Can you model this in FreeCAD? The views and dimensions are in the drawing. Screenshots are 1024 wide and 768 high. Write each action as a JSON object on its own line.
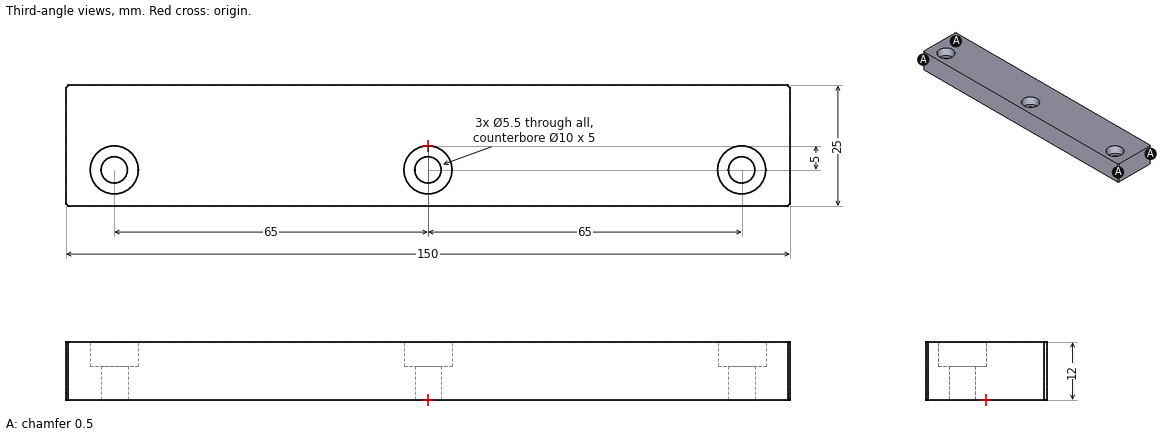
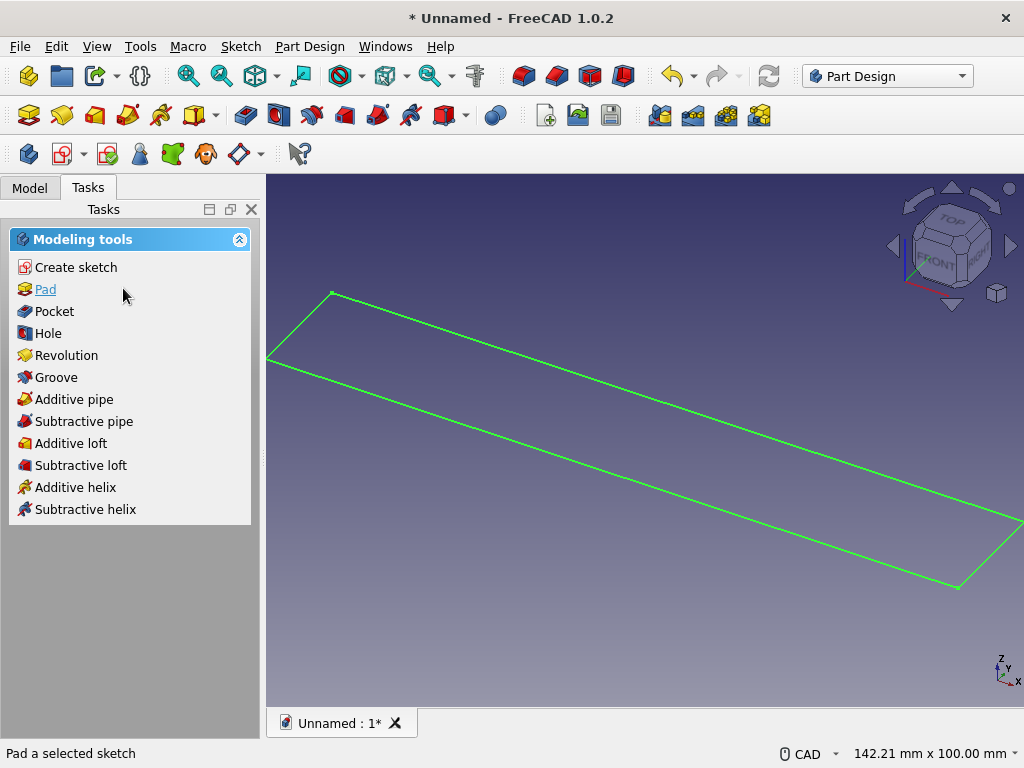
{"action": "left_click", "coordinate": [29, 116]}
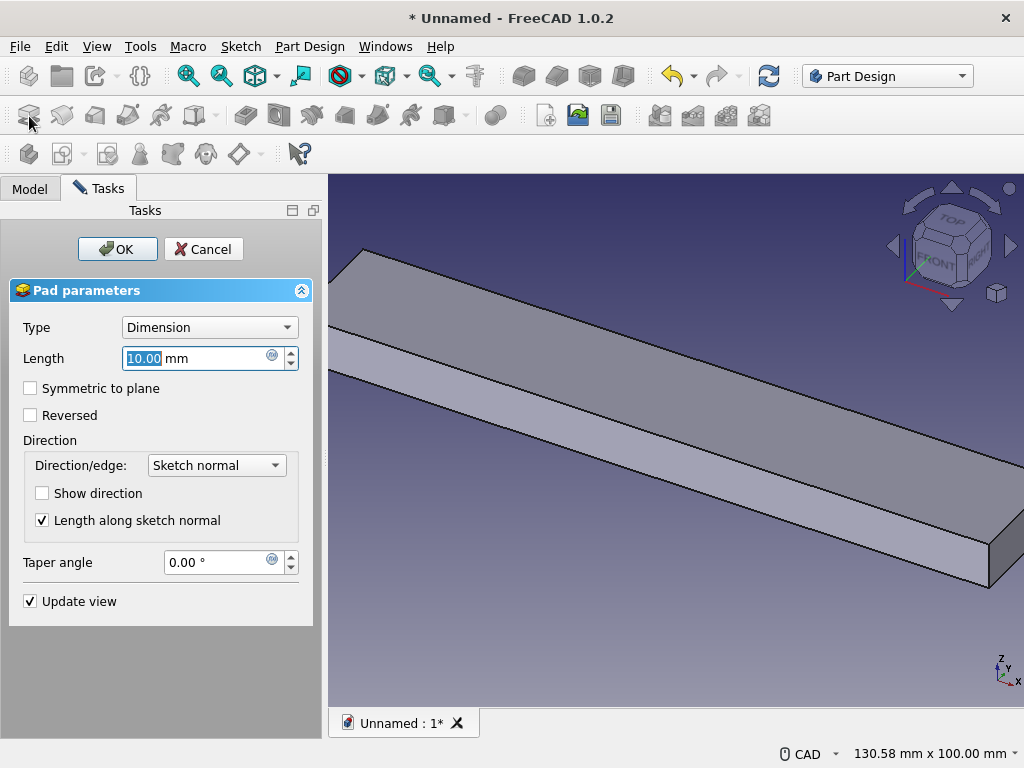
{"action": "type", "text": "12"}
{"action": "key", "text": "Tab"}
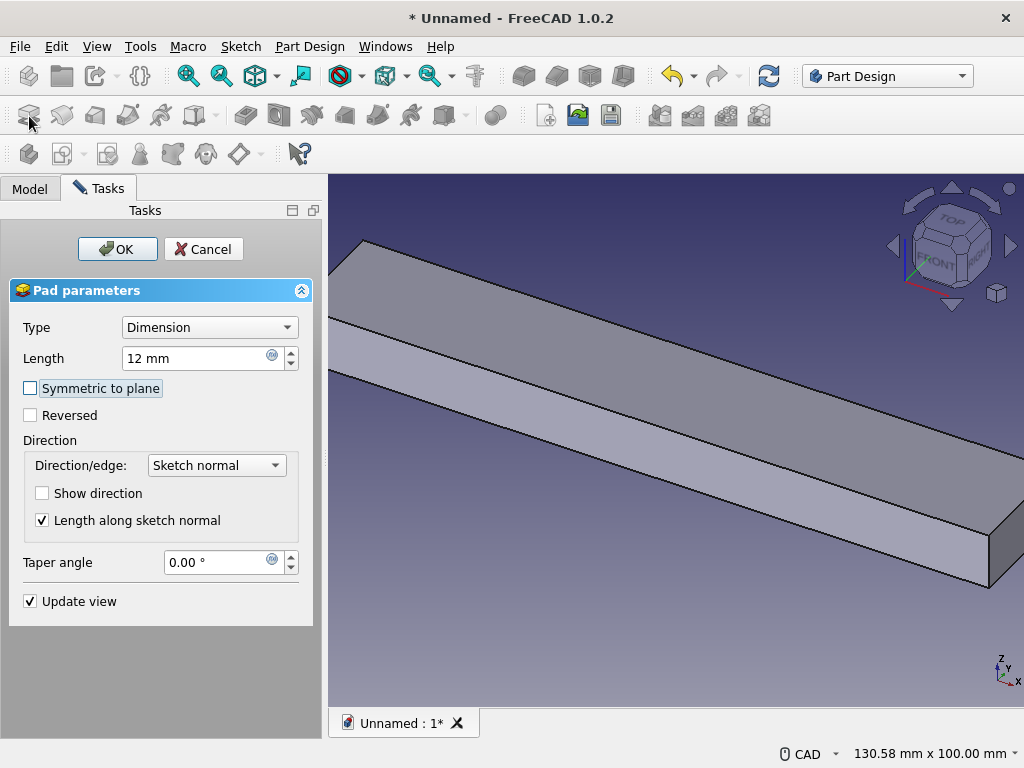
{"action": "left_click", "coordinate": [118, 249]}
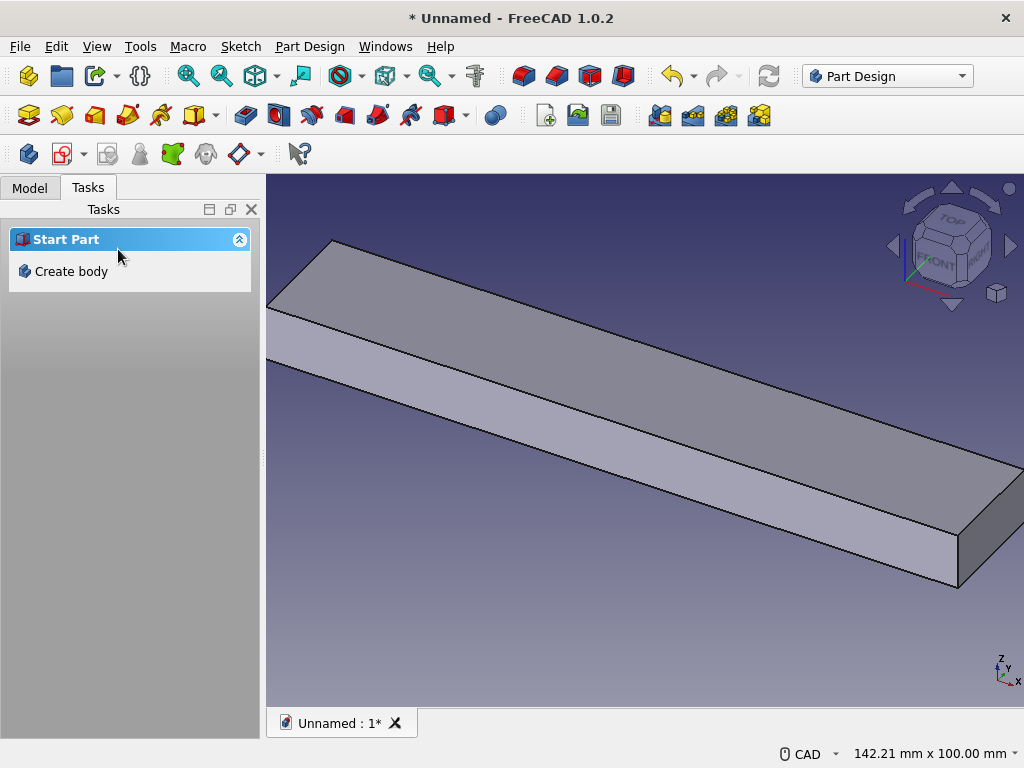
{"action": "left_click", "coordinate": [189, 76]}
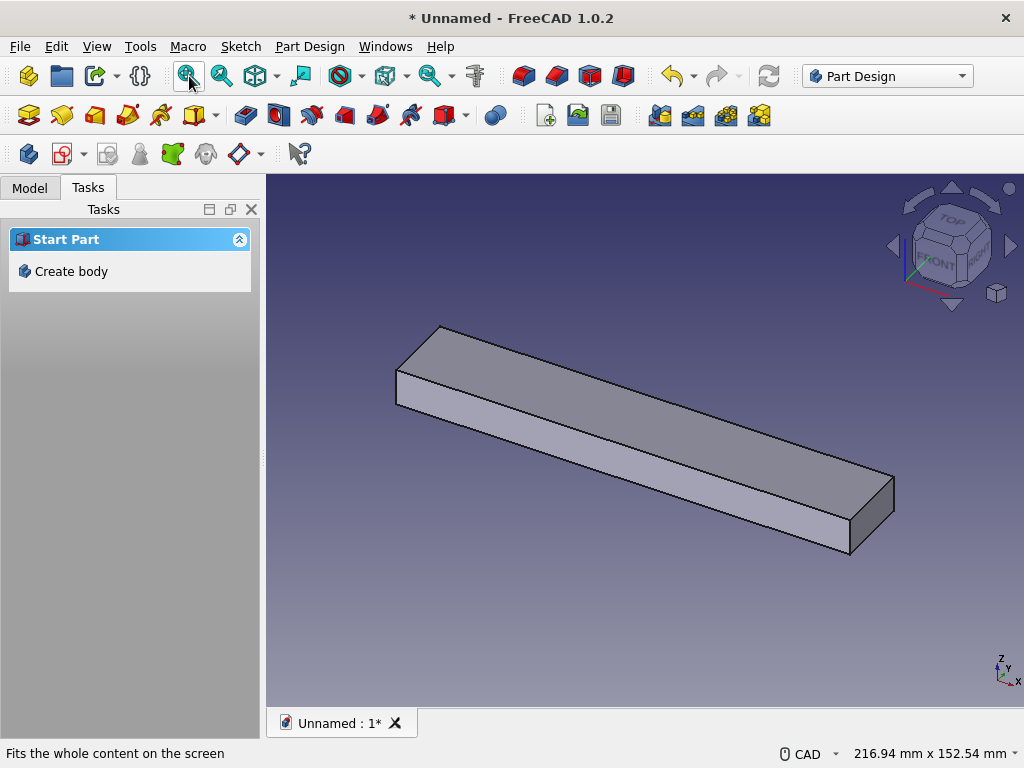
{"action": "left_click", "coordinate": [775, 465]}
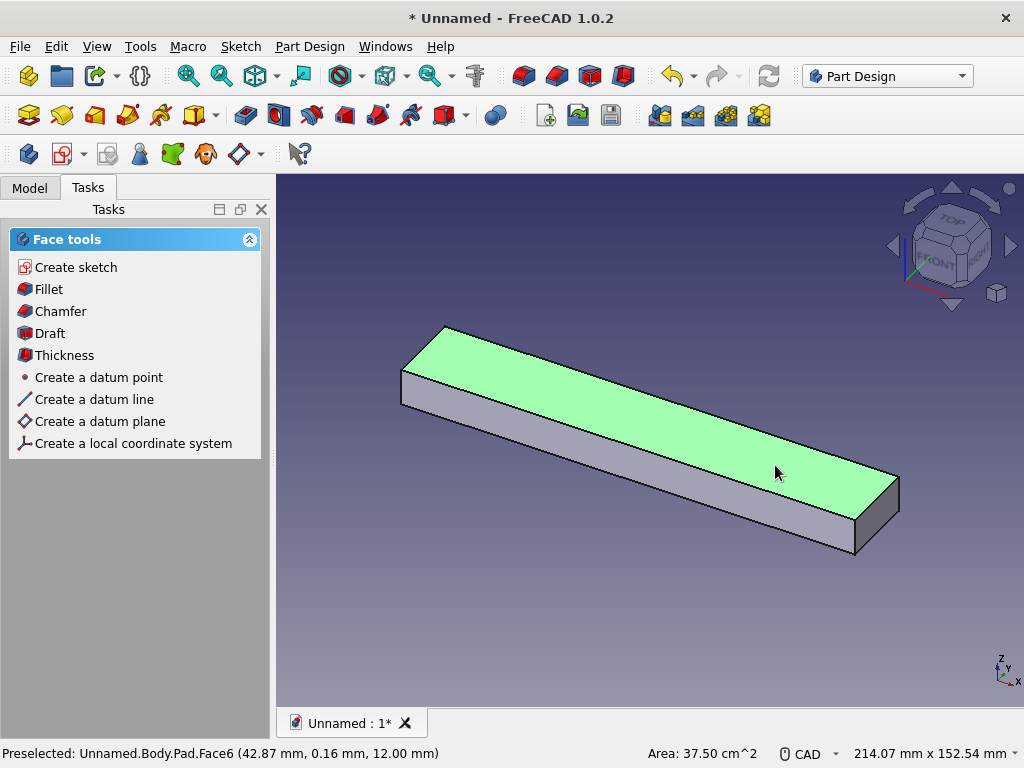
{"action": "left_click", "coordinate": [62, 154]}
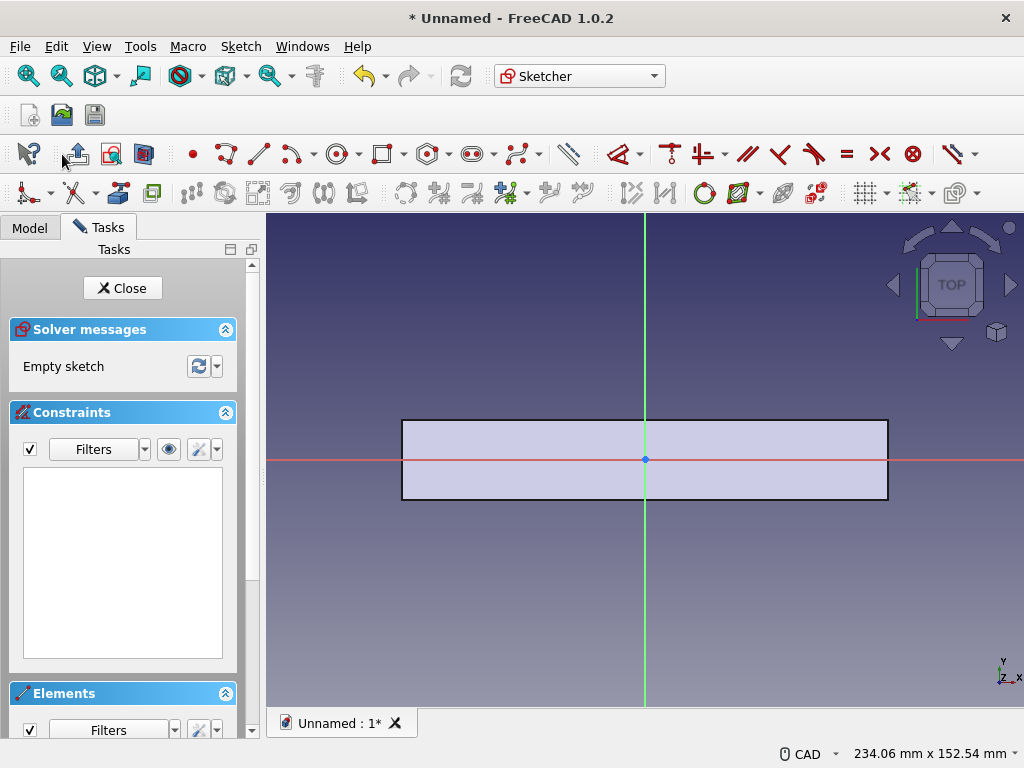
{"action": "scroll", "coordinate": [294, 403], "scroll_direction": "down", "scroll_amount": 1}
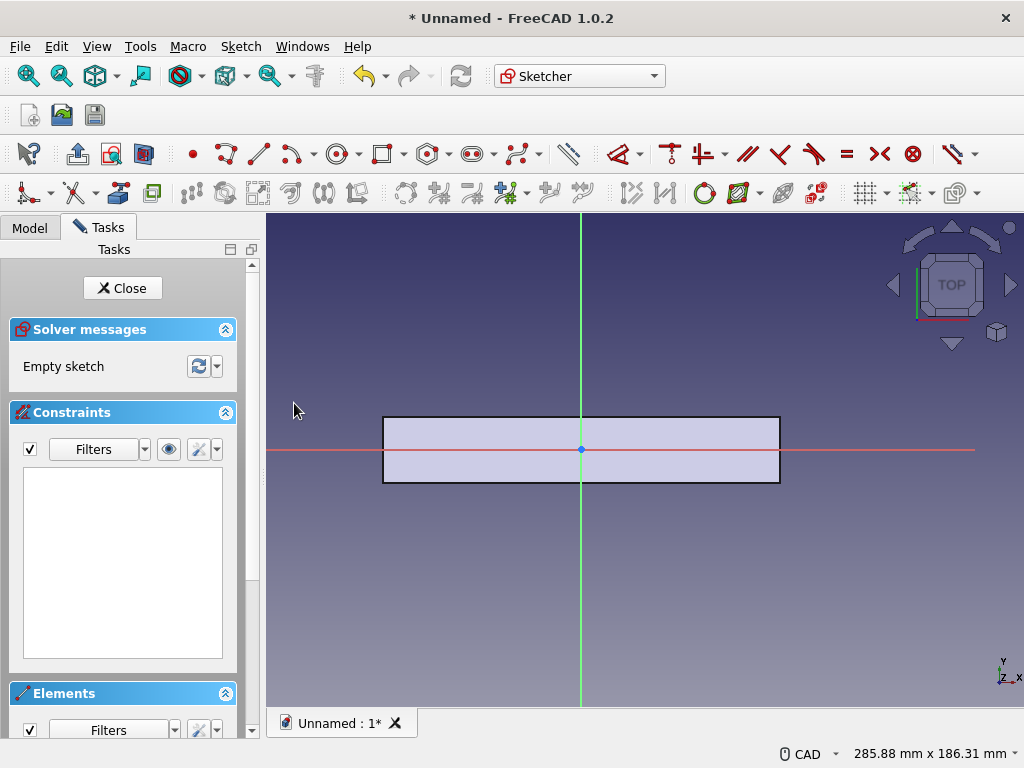
{"action": "left_click", "coordinate": [336, 154]}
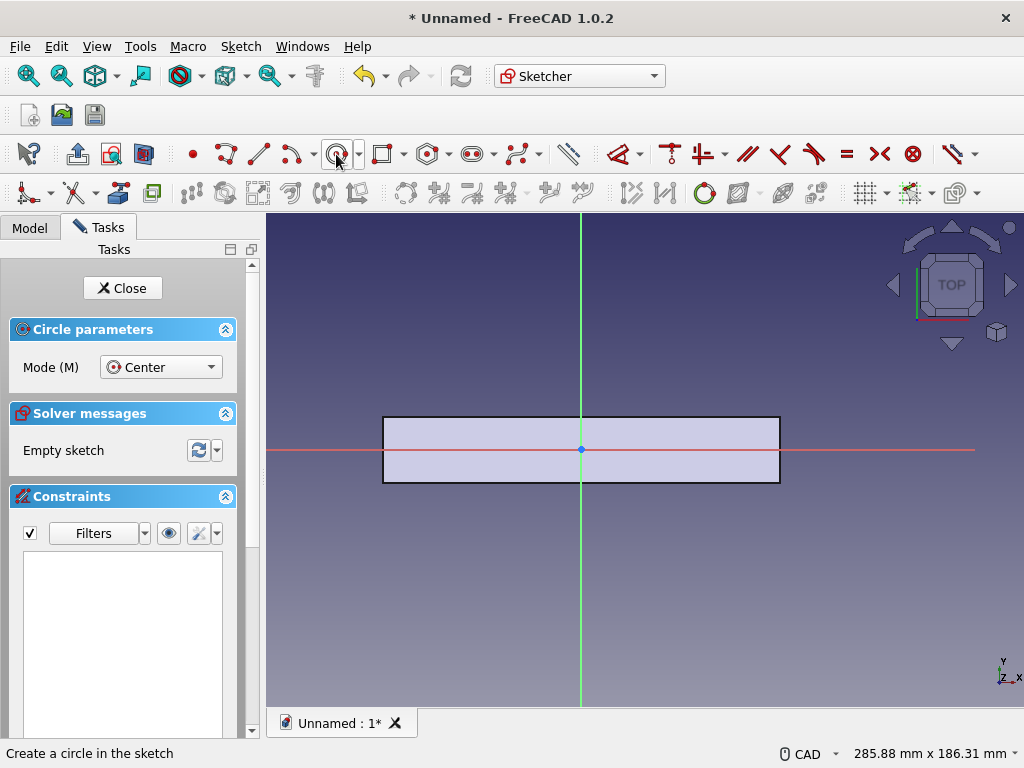
{"action": "scroll", "coordinate": [581, 463], "scroll_direction": "up", "scroll_amount": 6}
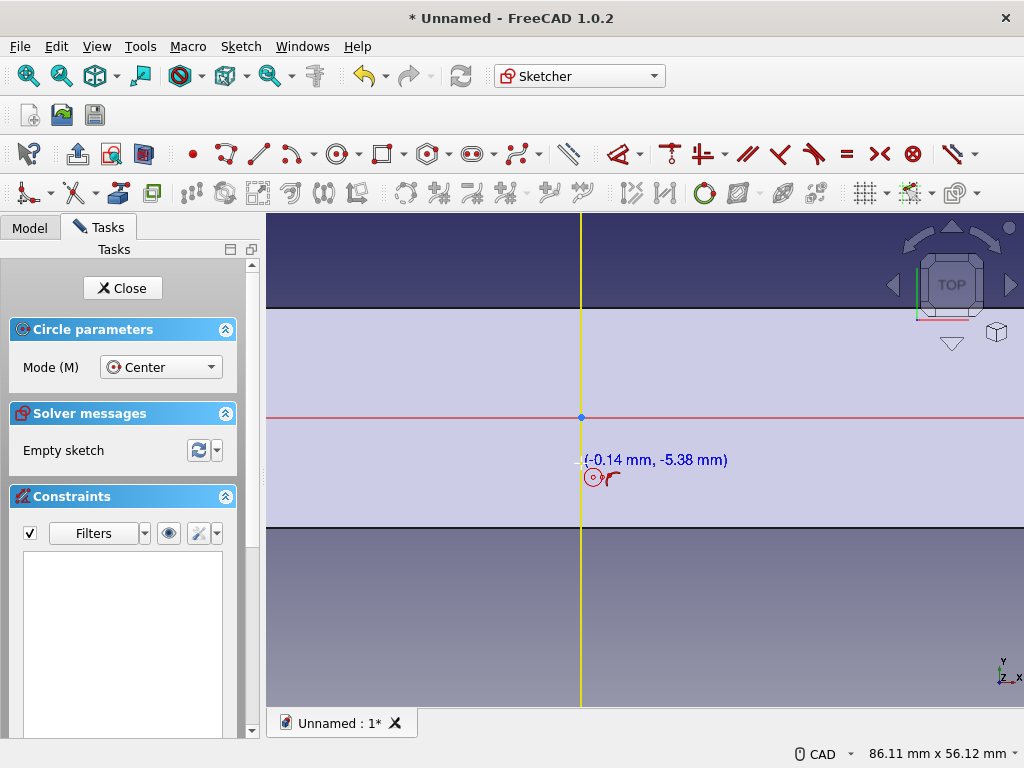
{"action": "left_click", "coordinate": [581, 462]}
{"action": "left_click", "coordinate": [598, 445]}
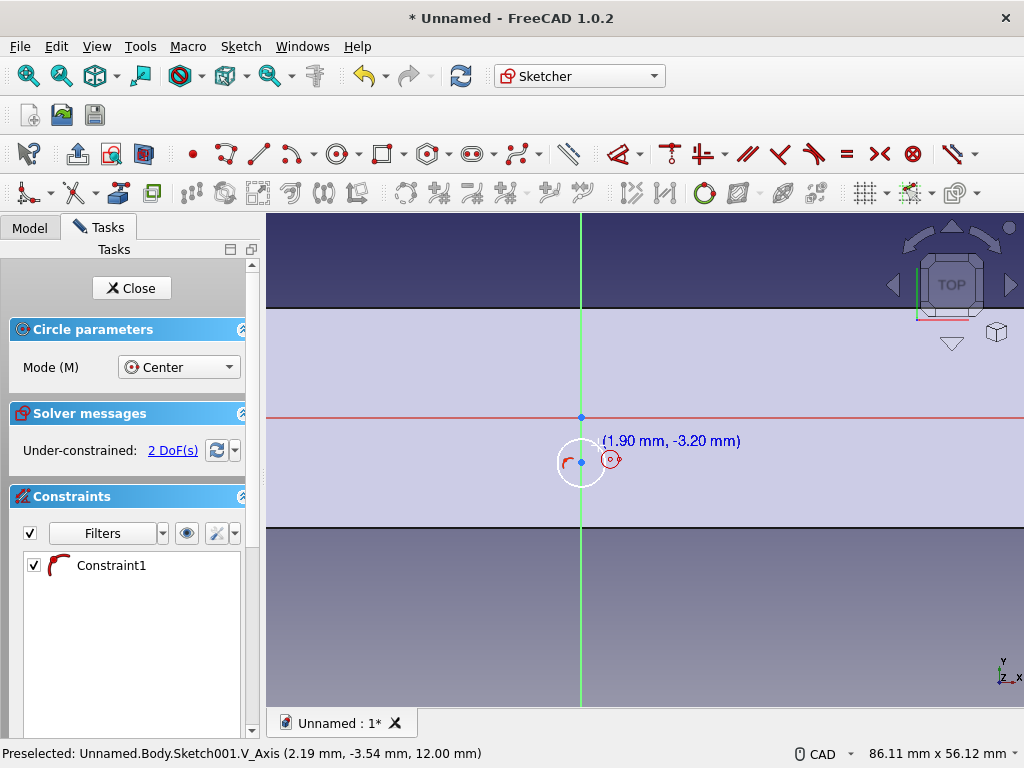
{"action": "scroll", "coordinate": [574, 465], "scroll_direction": "down", "scroll_amount": 5}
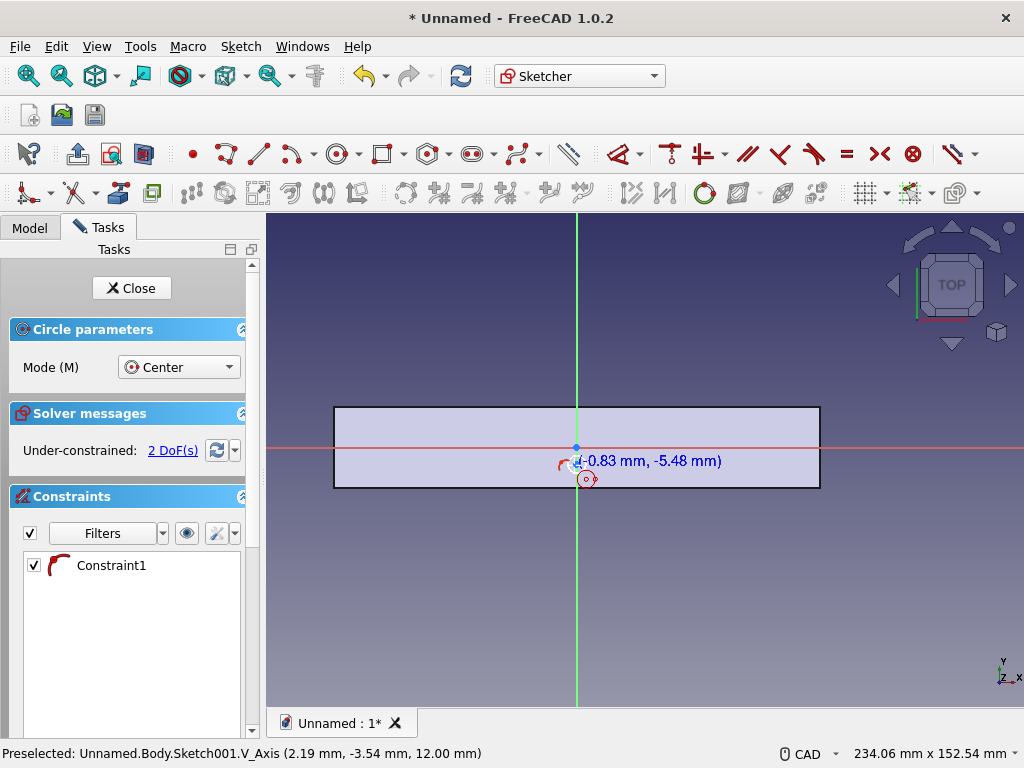
{"action": "scroll", "coordinate": [366, 464], "scroll_direction": "up", "scroll_amount": 5}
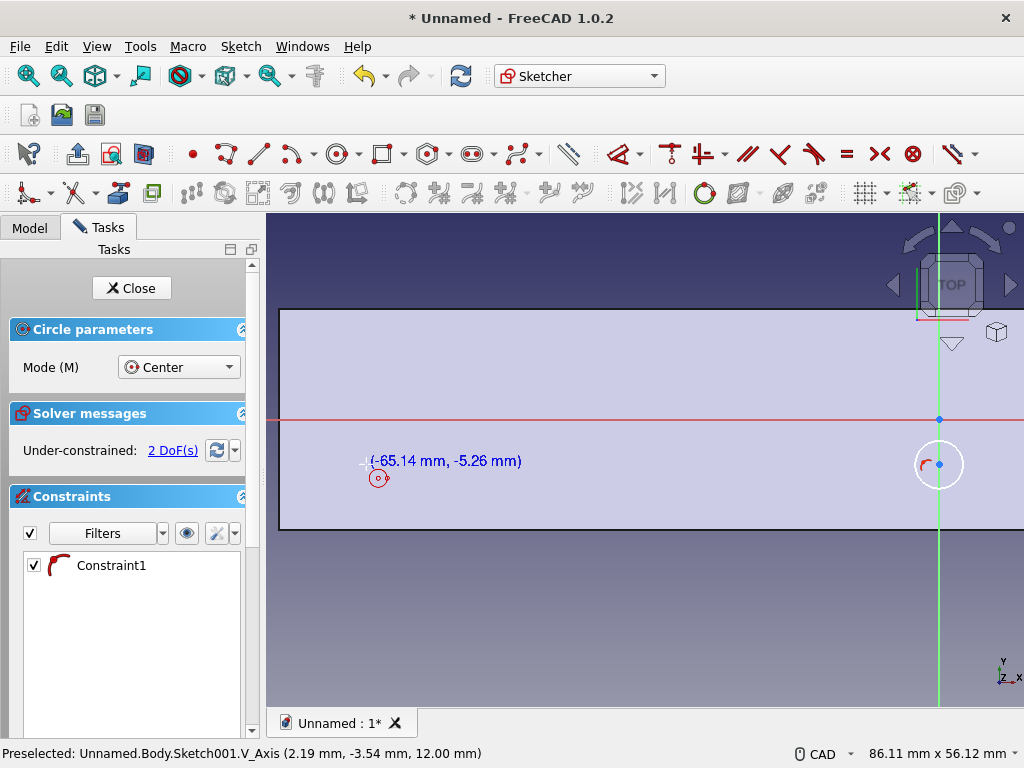
{"action": "left_click", "coordinate": [367, 464]}
{"action": "left_click", "coordinate": [384, 446]}